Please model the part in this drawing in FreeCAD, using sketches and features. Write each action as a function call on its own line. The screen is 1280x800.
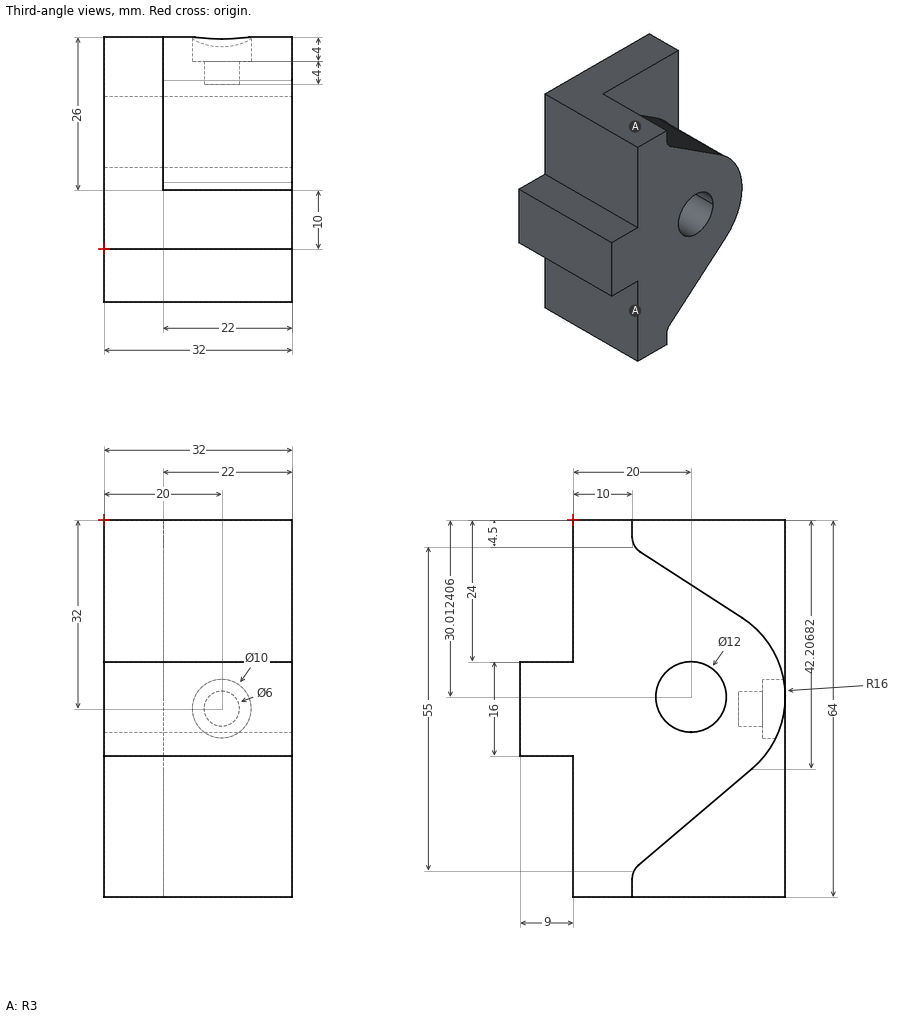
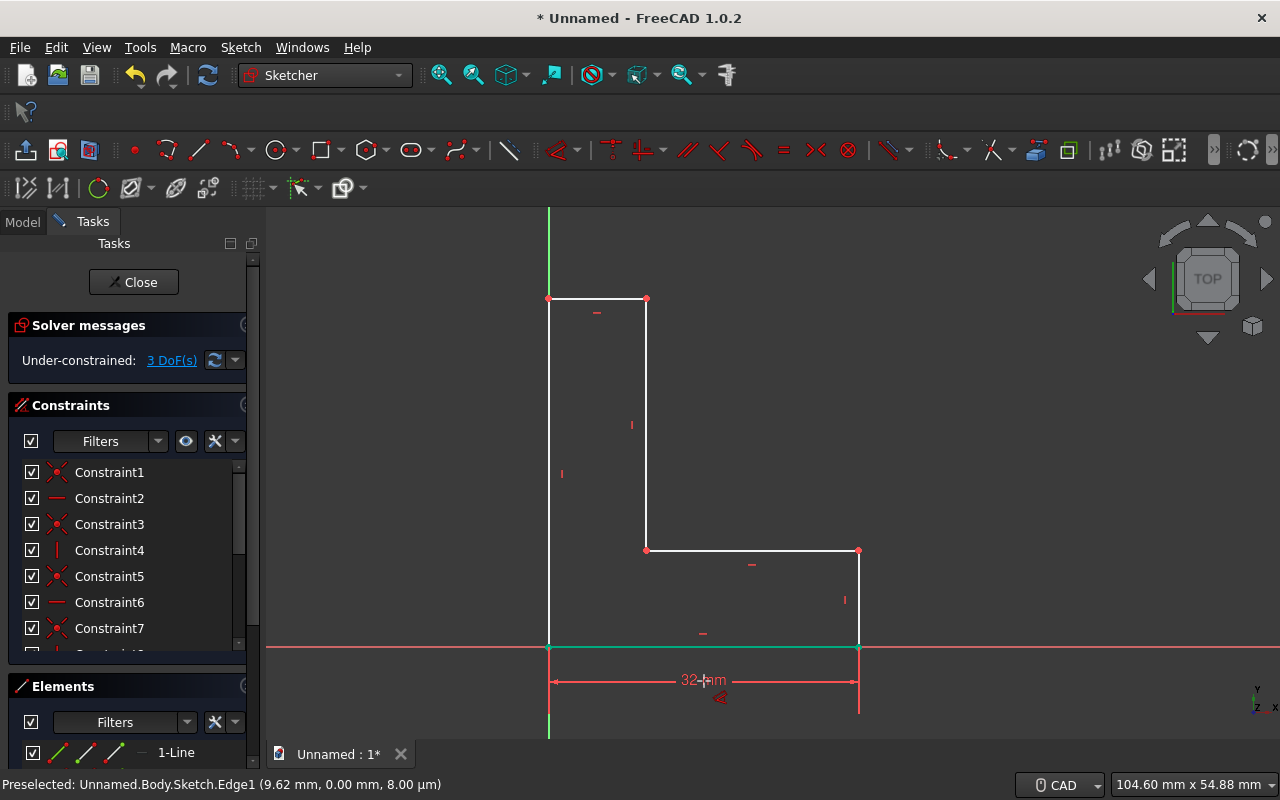
click(859, 618)
click(893, 599)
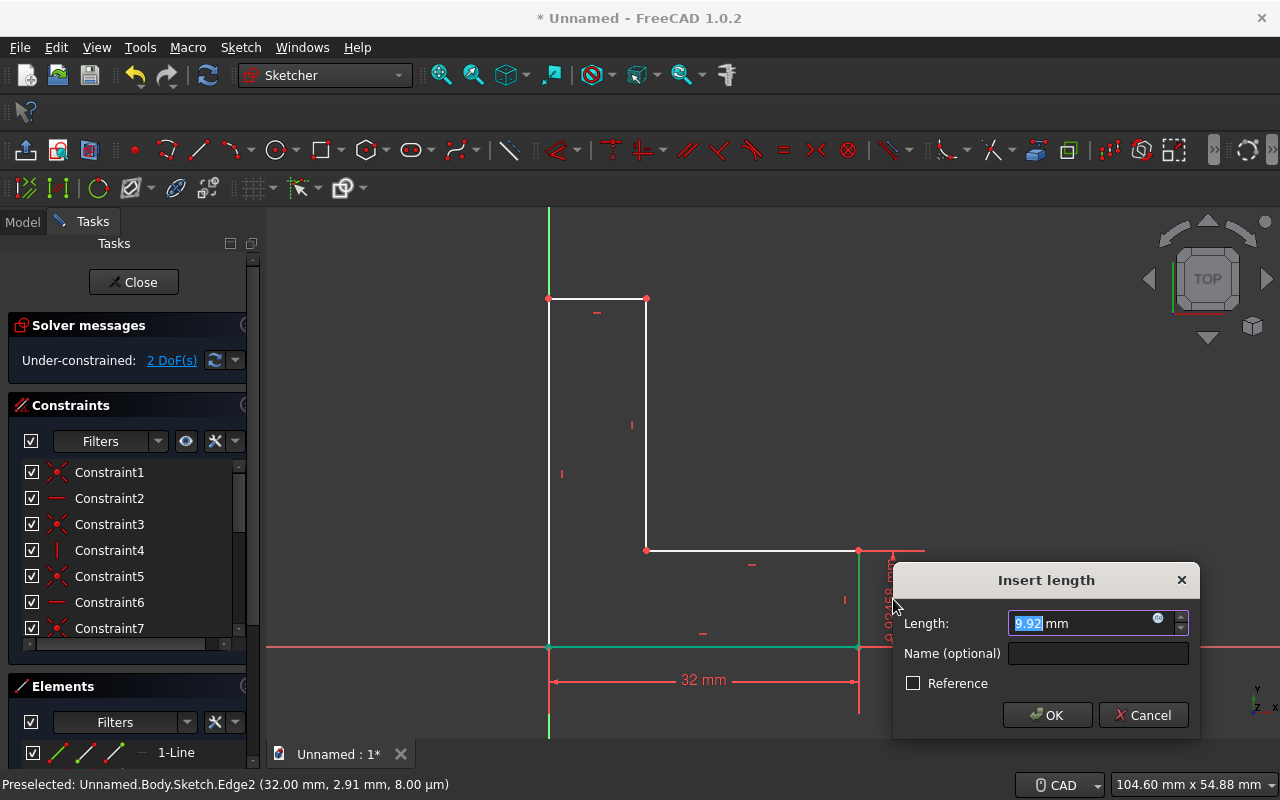
text(10)
key(Return)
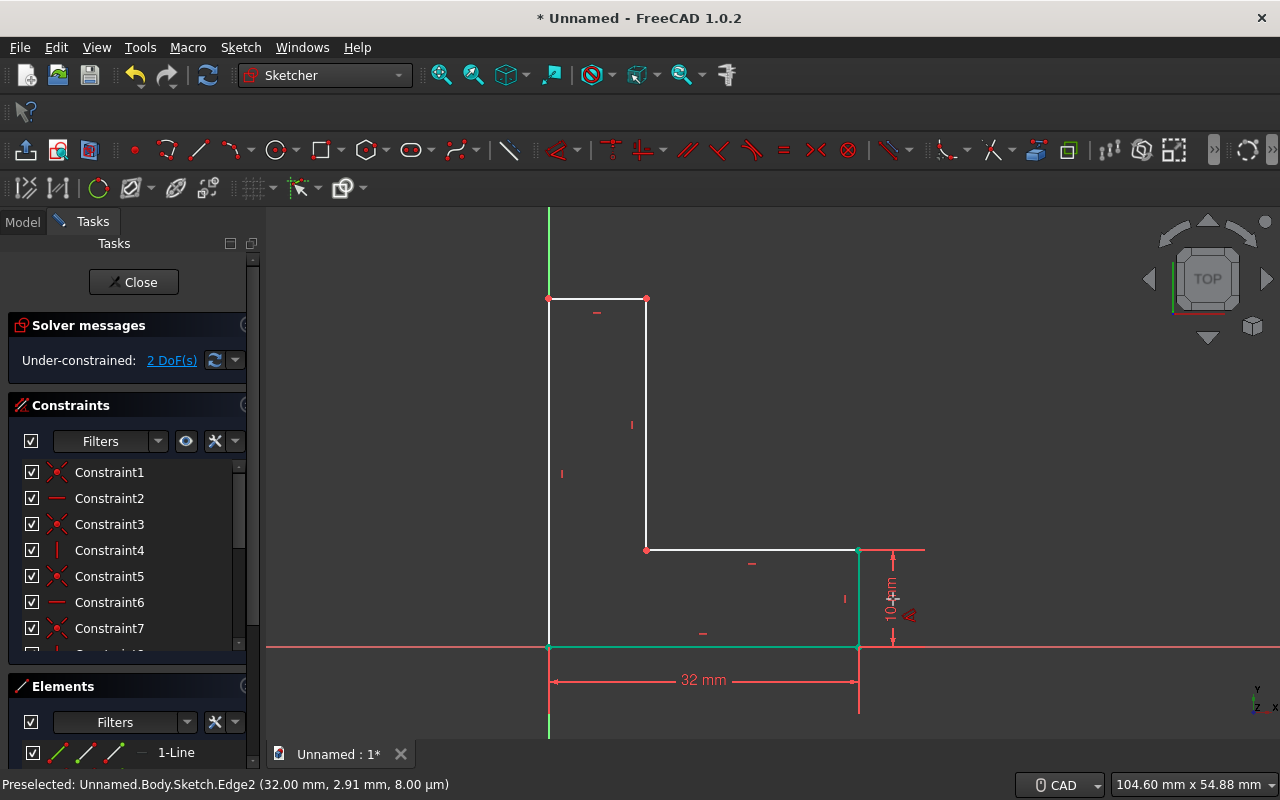
click(795, 550)
click(752, 584)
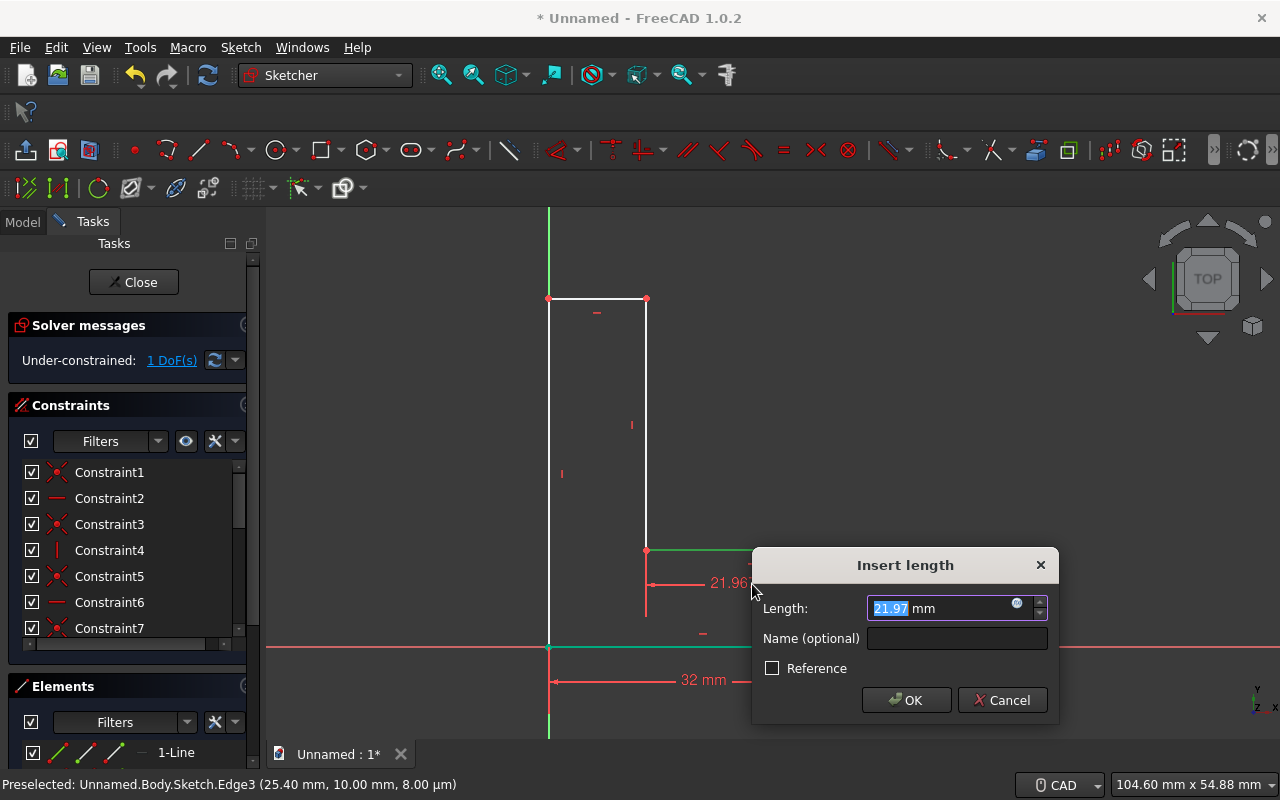
text(22)
key(Return)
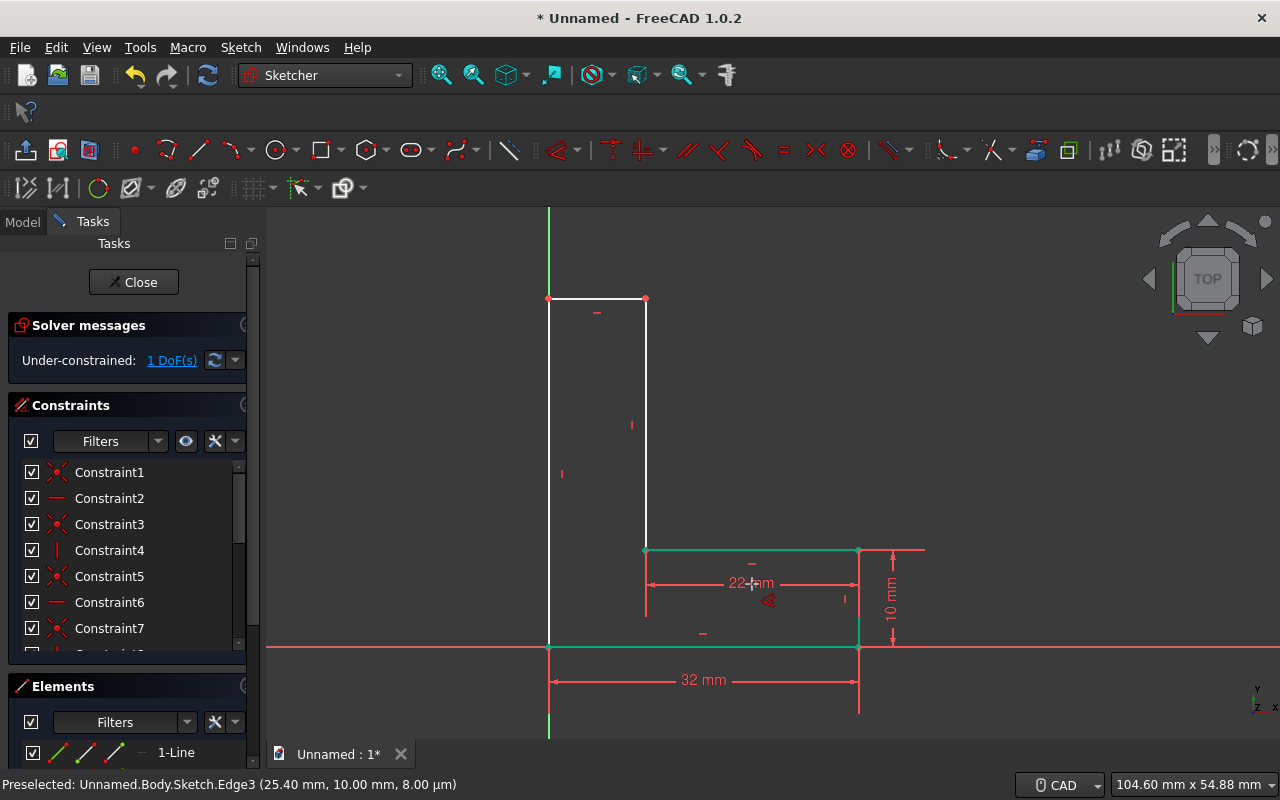
click(646, 475)
click(612, 425)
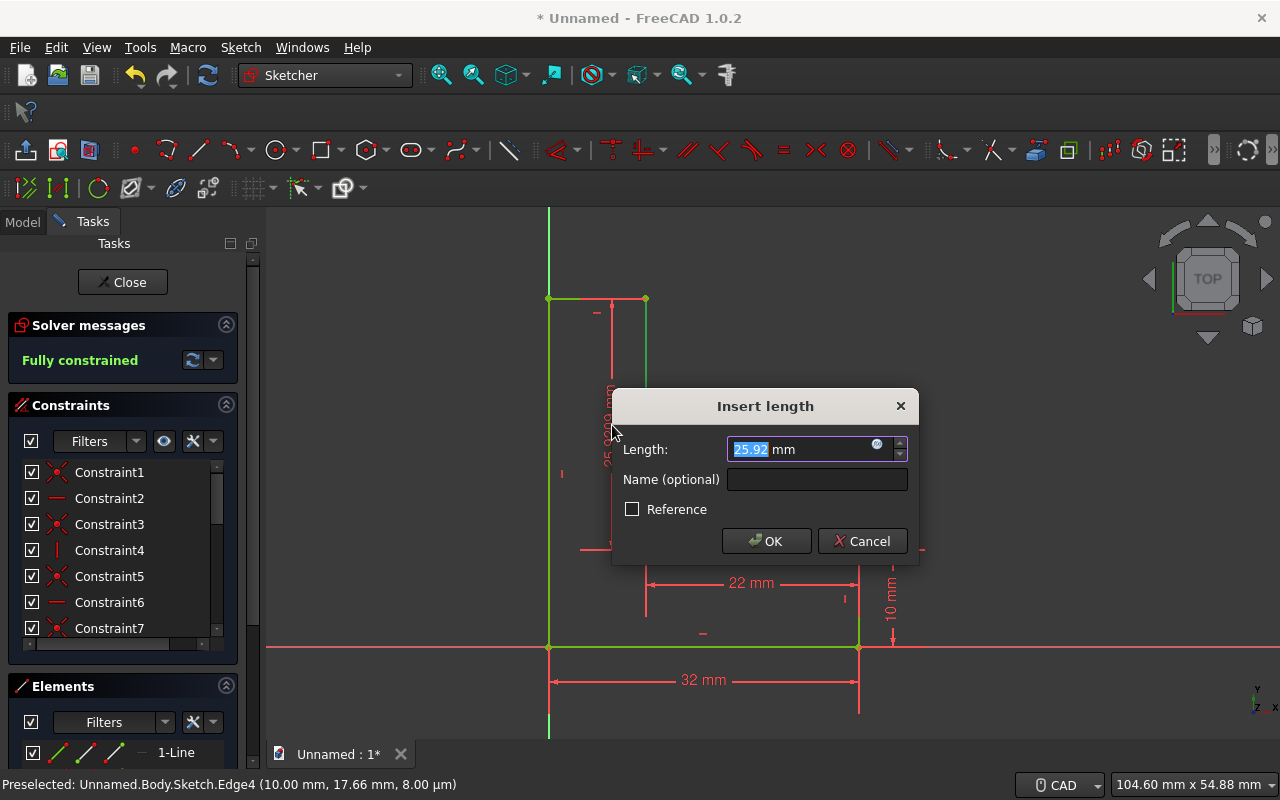
text(26)
key(Return)
key(Escape)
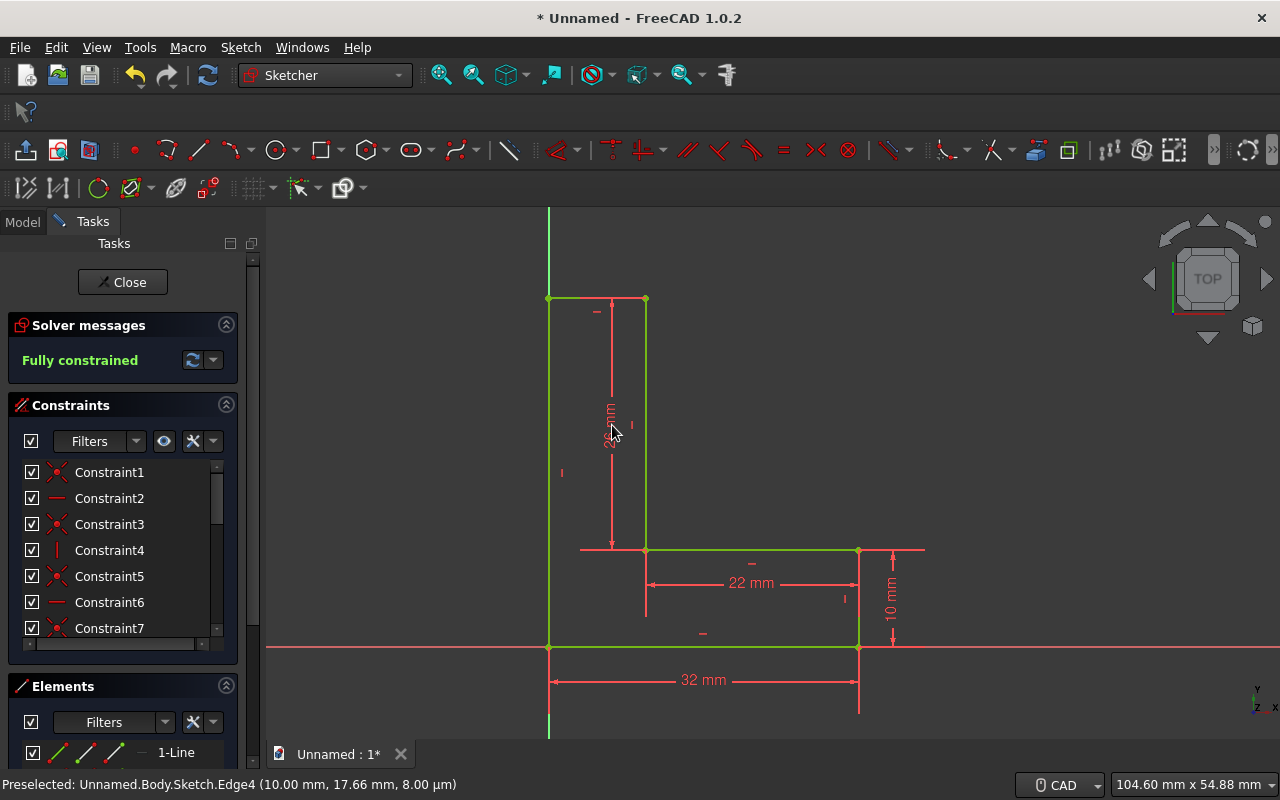
click(123, 282)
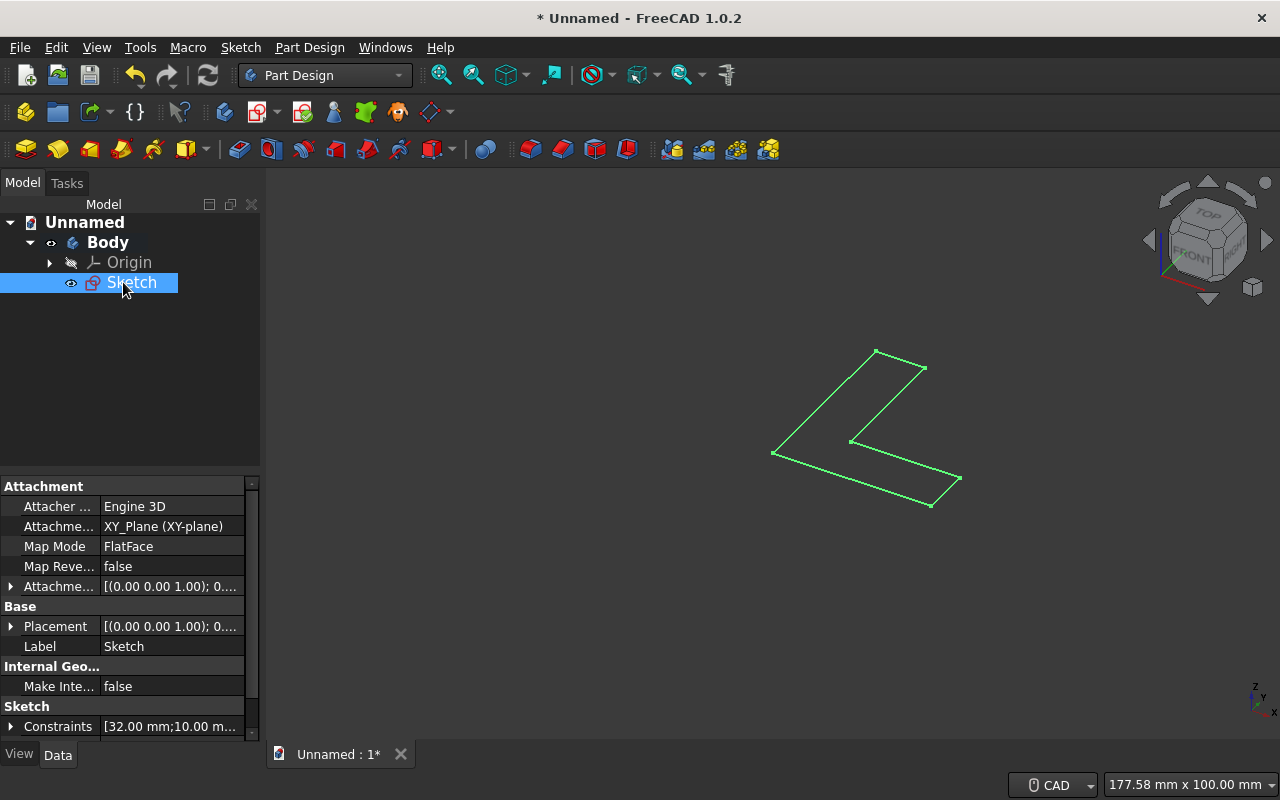
click(26, 150)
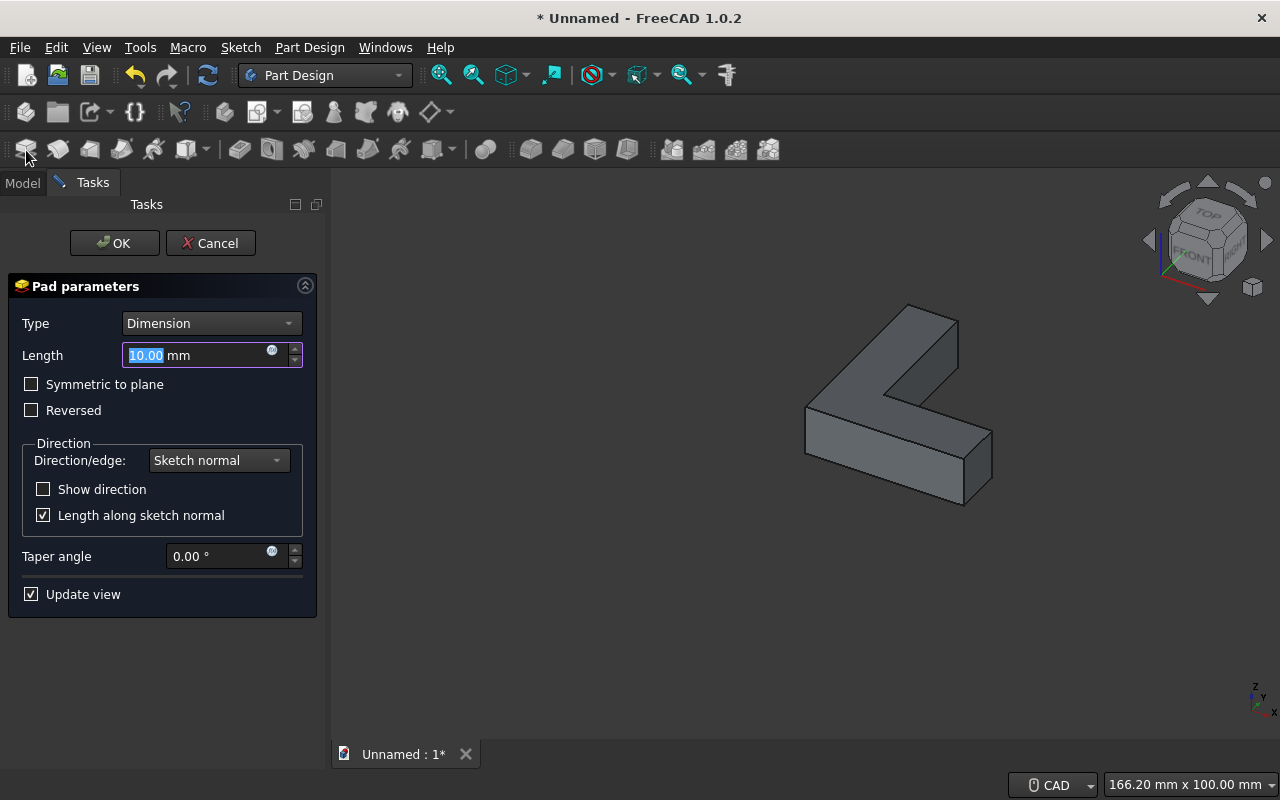
text(64)
key(Tab)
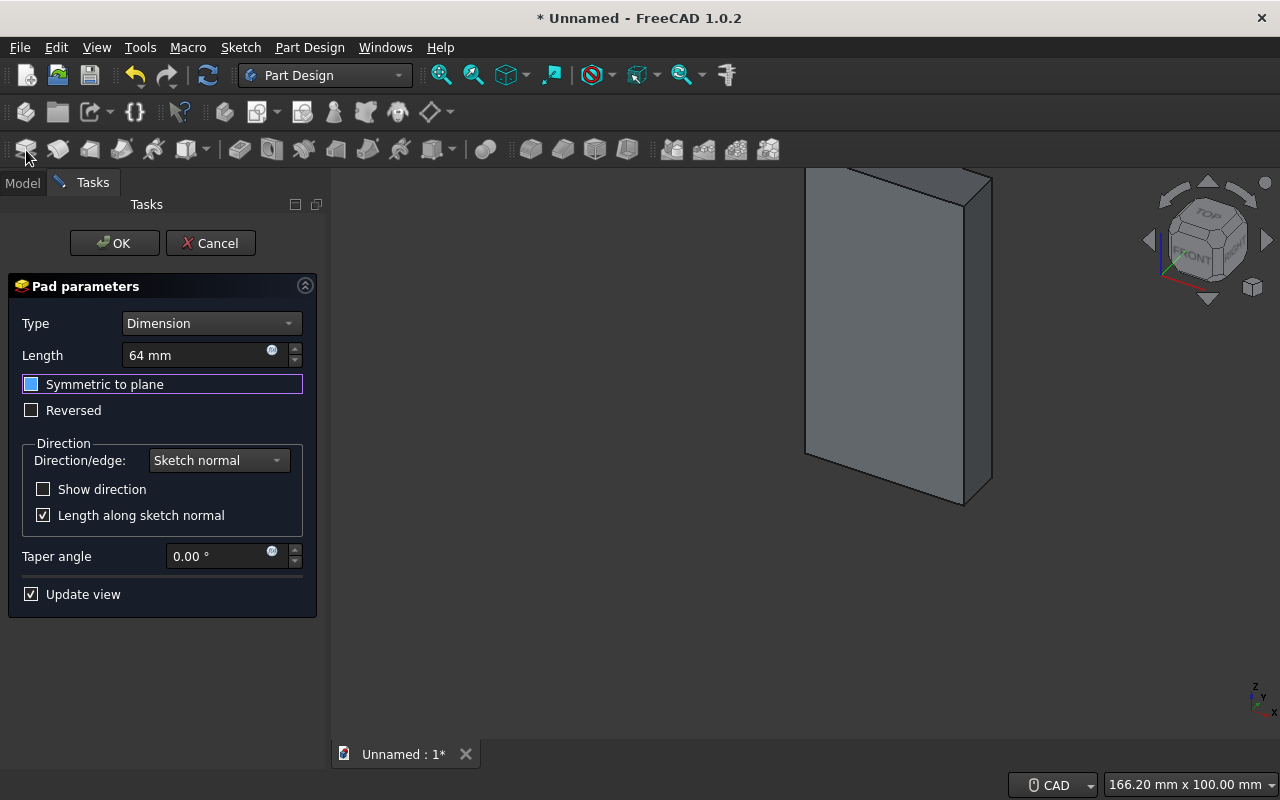
click(30, 410)